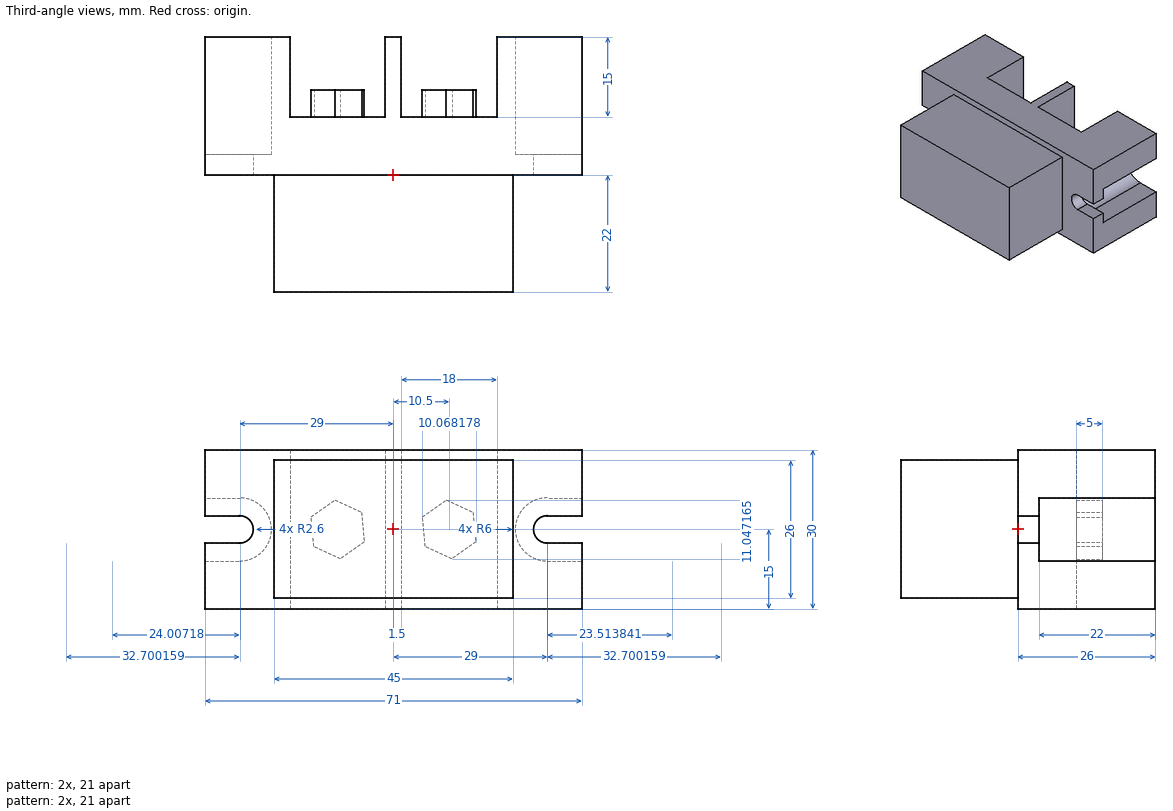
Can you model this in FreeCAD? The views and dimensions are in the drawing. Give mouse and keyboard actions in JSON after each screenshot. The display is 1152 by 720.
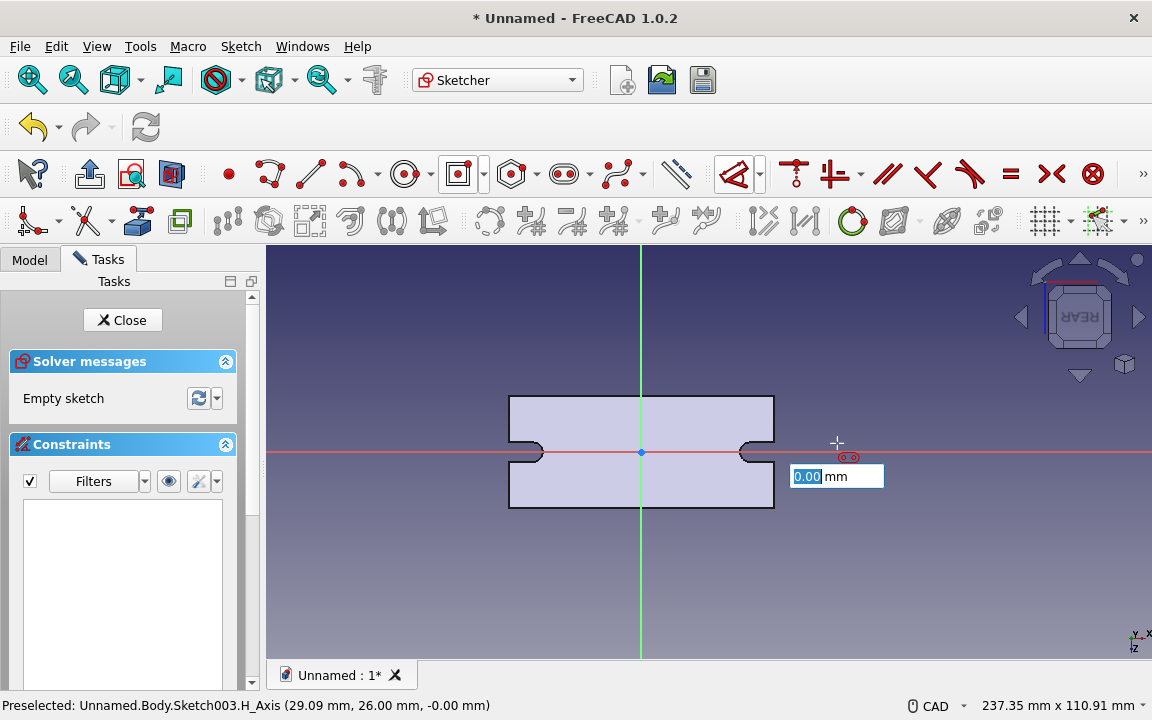
{"action": "left_click", "coordinate": [794, 430]}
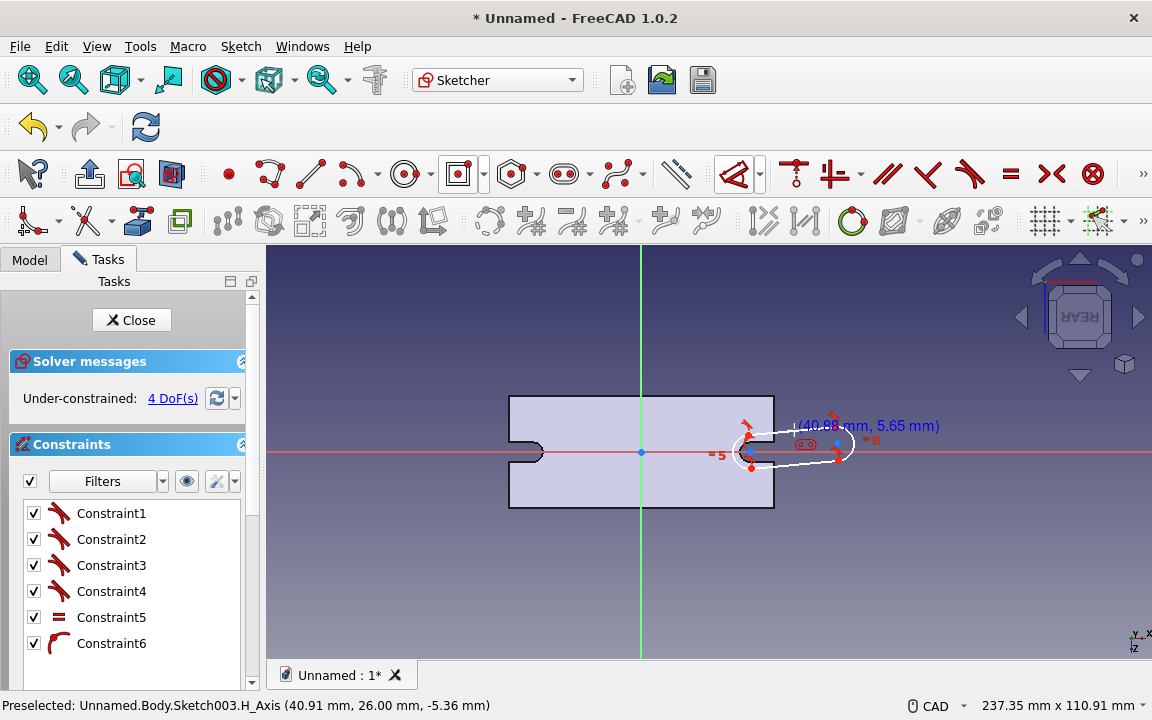
{"action": "left_click", "coordinate": [444, 452]}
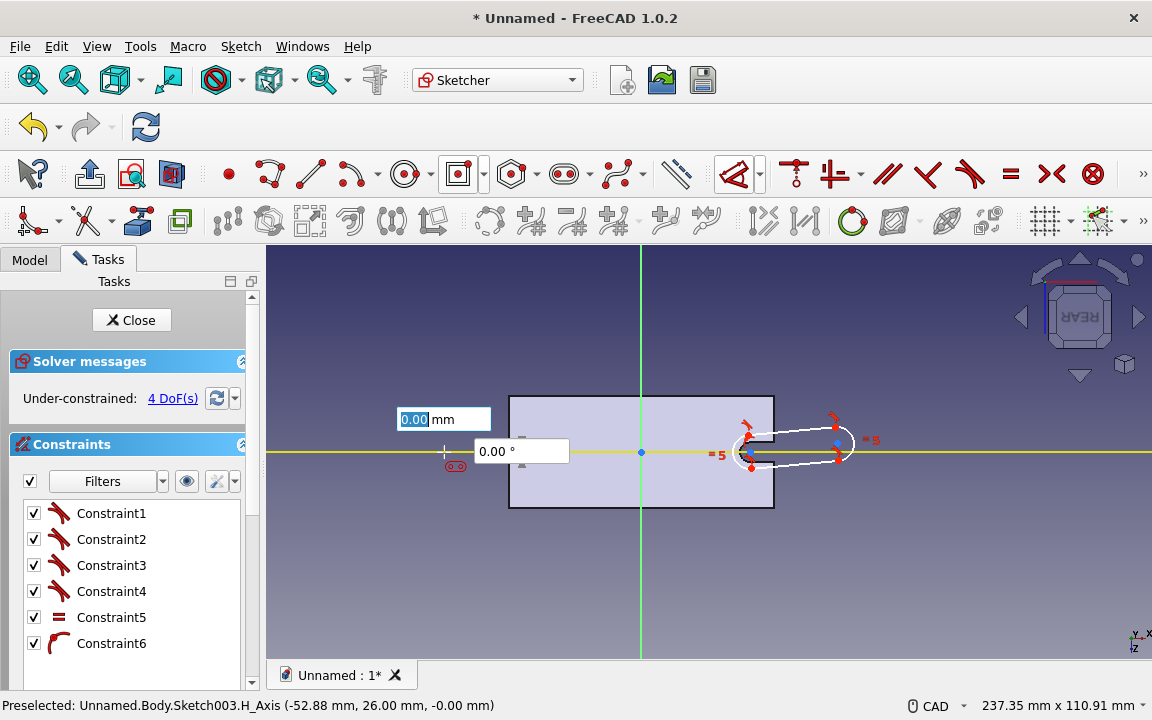
{"action": "left_click", "coordinate": [533, 443]}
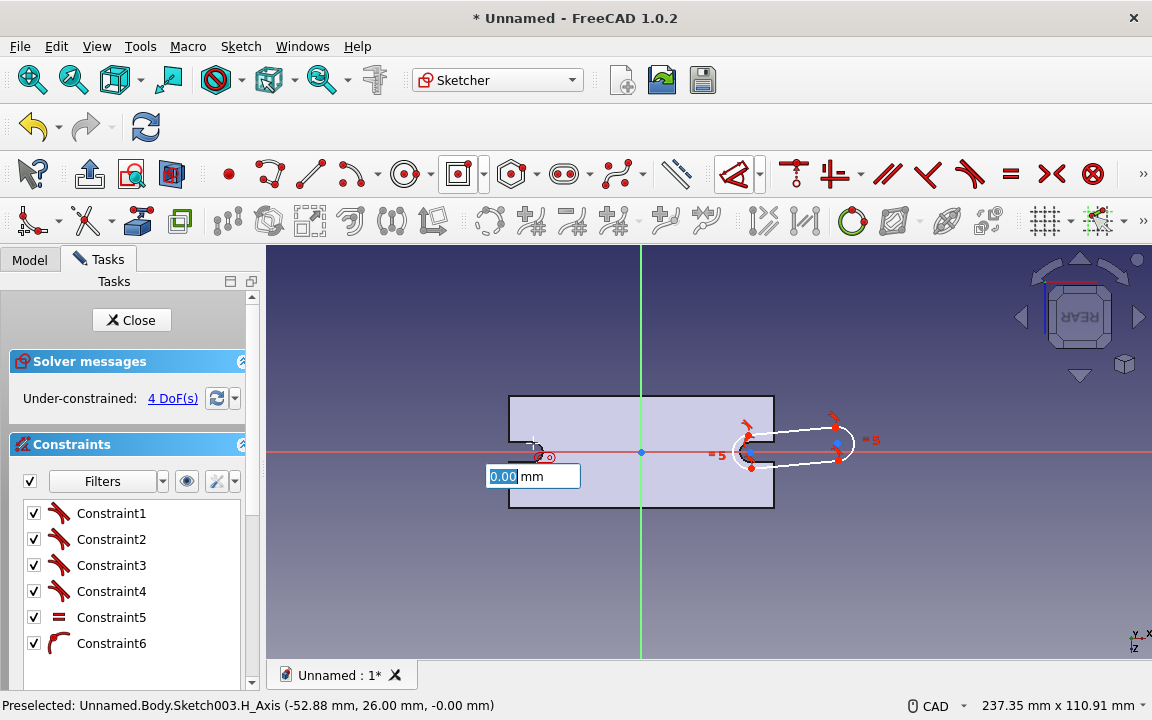
{"action": "left_click", "coordinate": [488, 474]}
{"action": "key", "text": "Escape"}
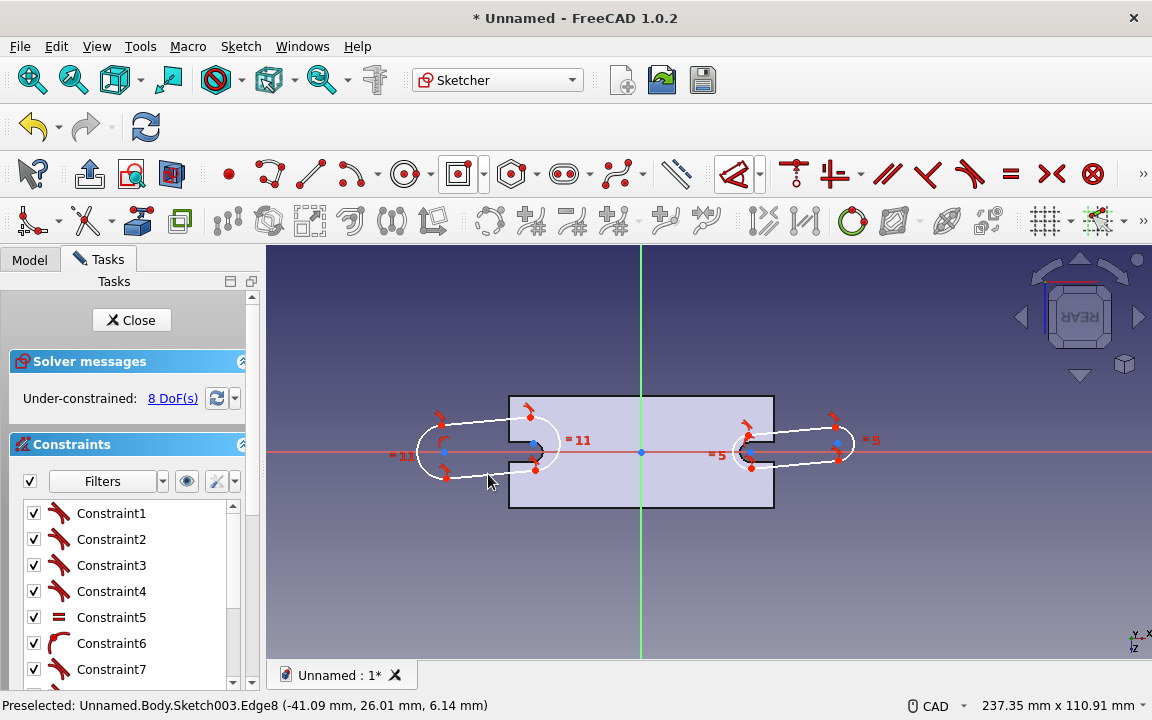
{"action": "left_click", "coordinate": [775, 433]}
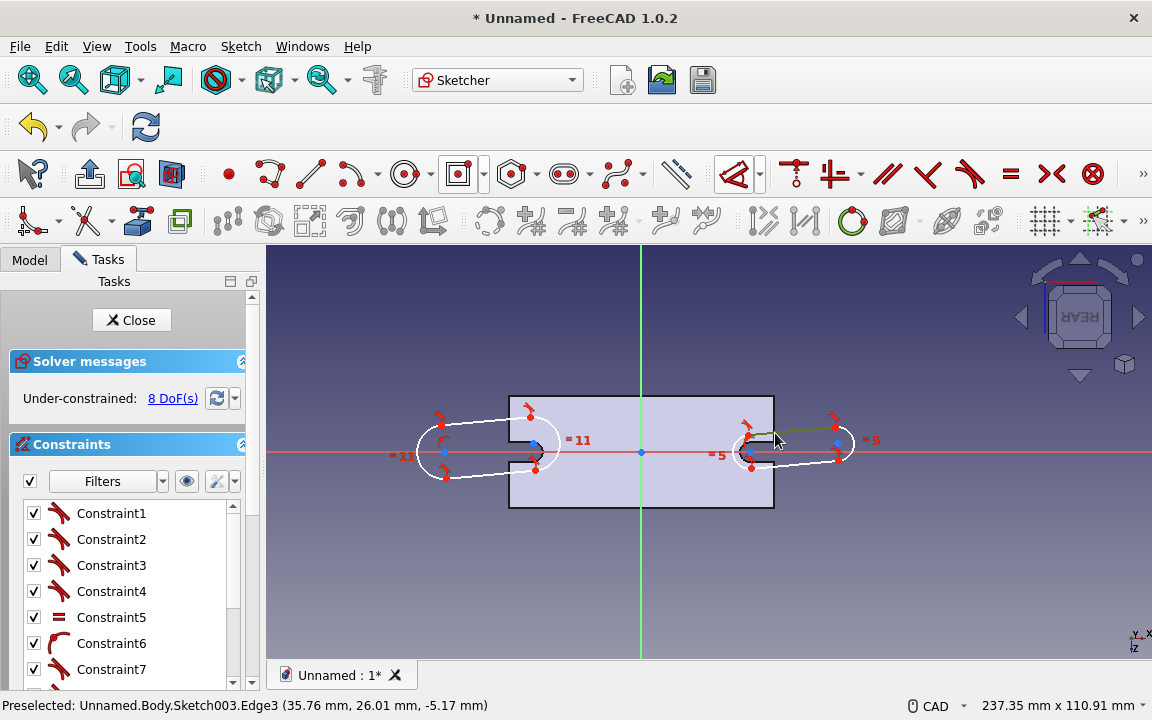
{"action": "left_click", "coordinate": [860, 174]}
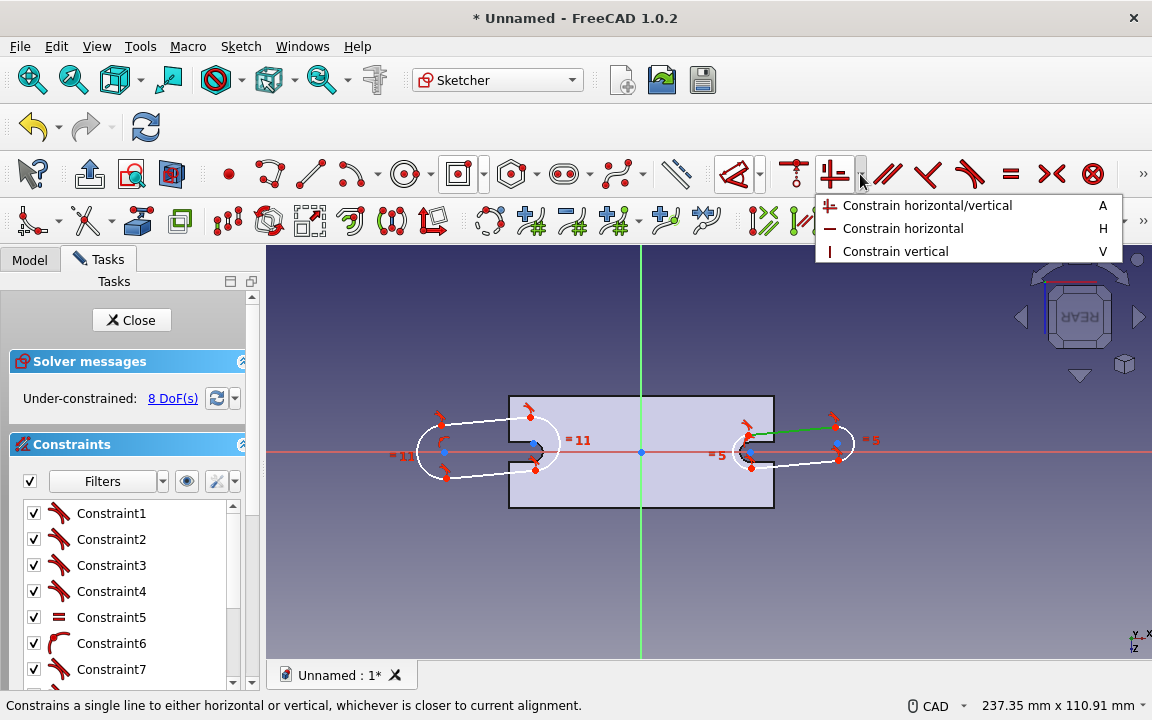
{"action": "left_click", "coordinate": [969, 228]}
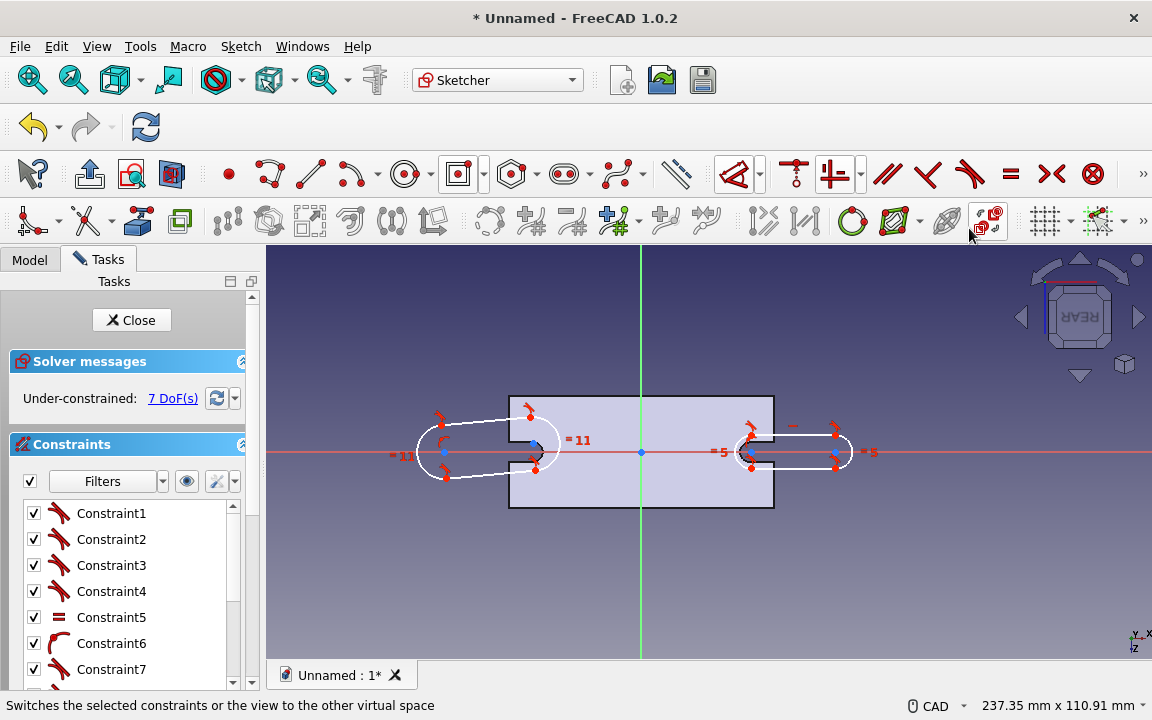
{"action": "left_click", "coordinate": [468, 423]}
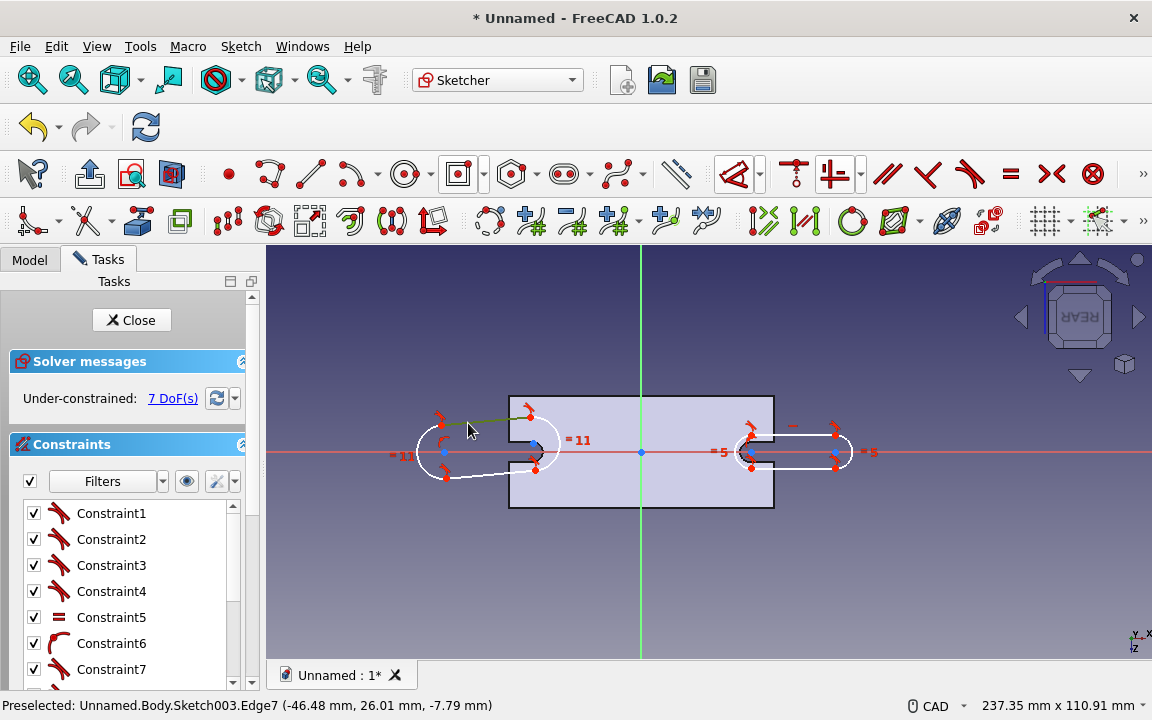
{"action": "left_click", "coordinate": [860, 174]}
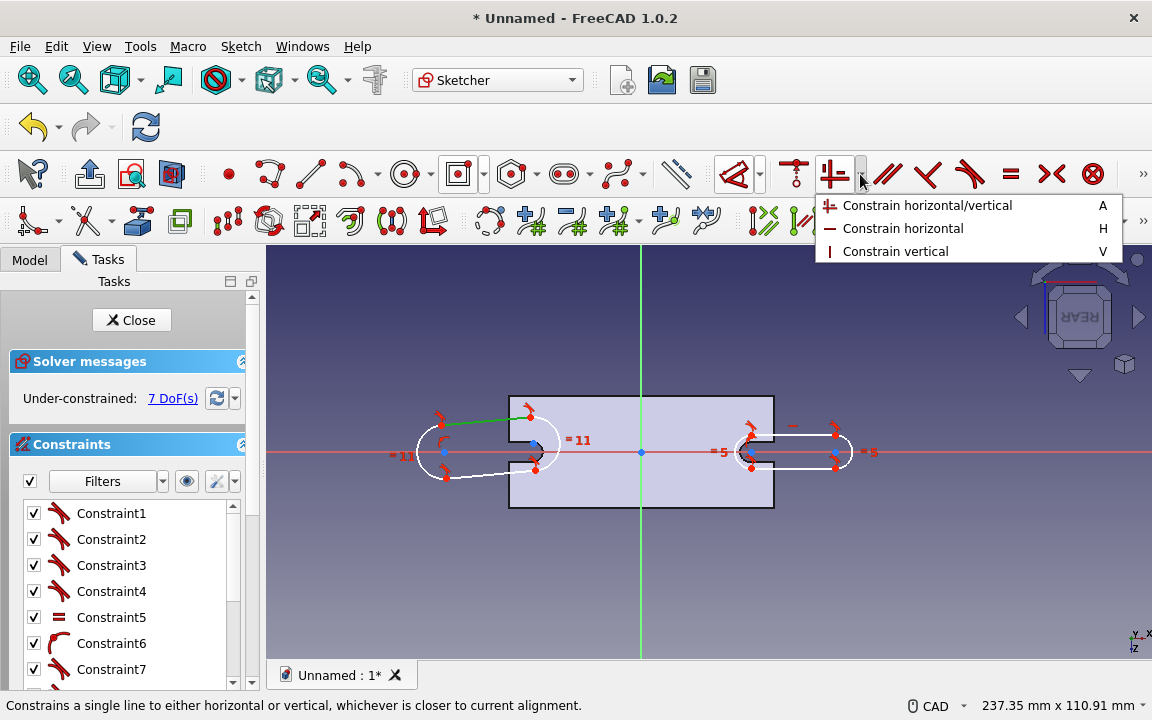
{"action": "left_click", "coordinate": [969, 228]}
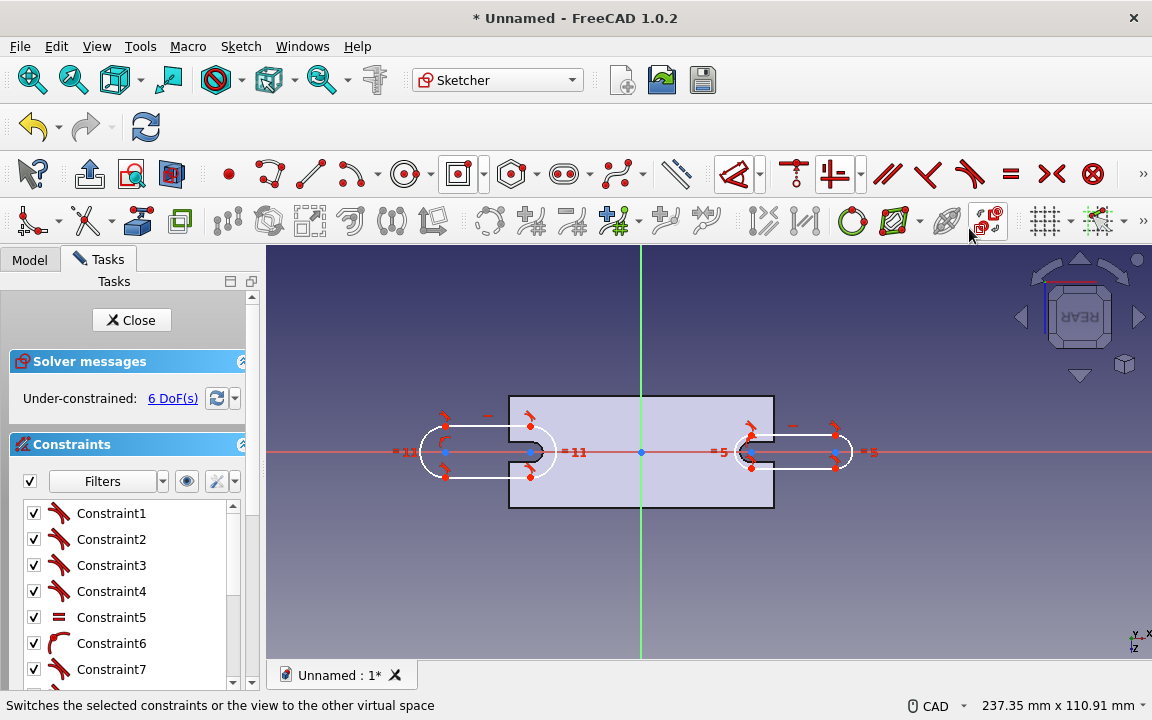
{"action": "scroll", "coordinate": [738, 442], "scroll_direction": "up", "scroll_amount": 2}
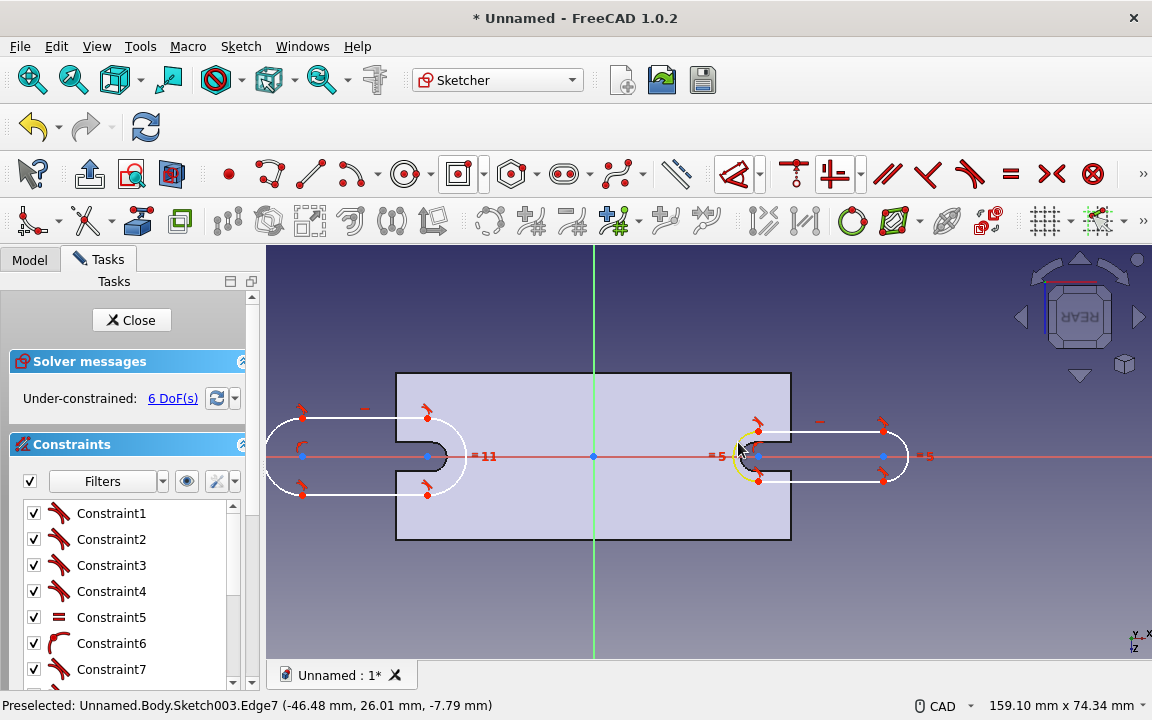
{"action": "left_click", "coordinate": [738, 442]}